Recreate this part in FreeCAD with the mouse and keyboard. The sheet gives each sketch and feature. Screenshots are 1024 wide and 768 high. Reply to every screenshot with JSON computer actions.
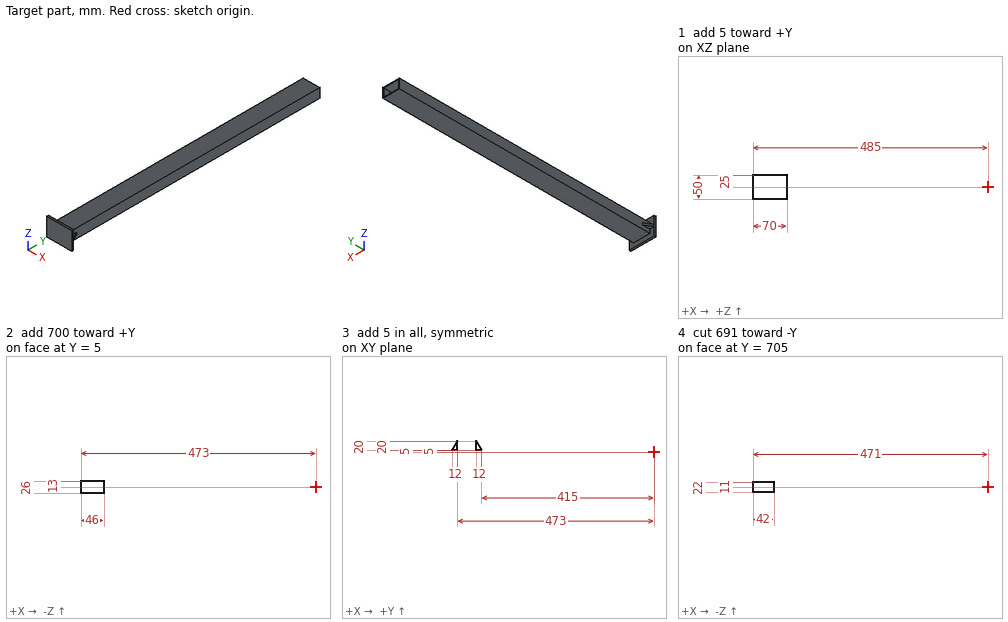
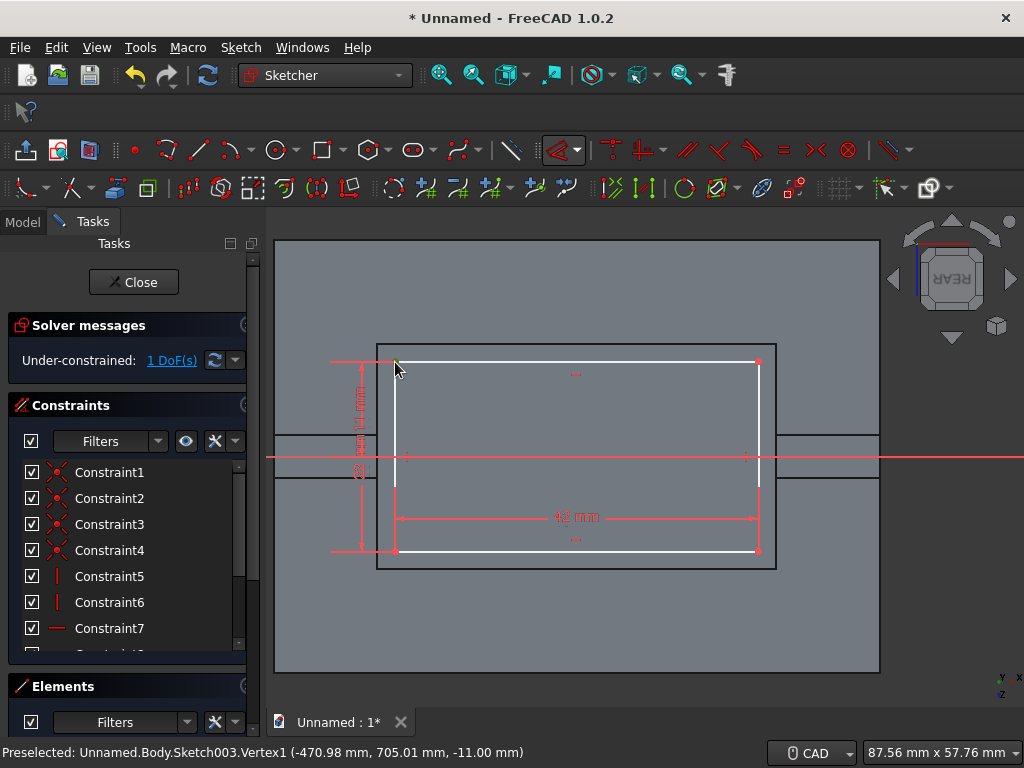
{"action": "key", "text": "l"}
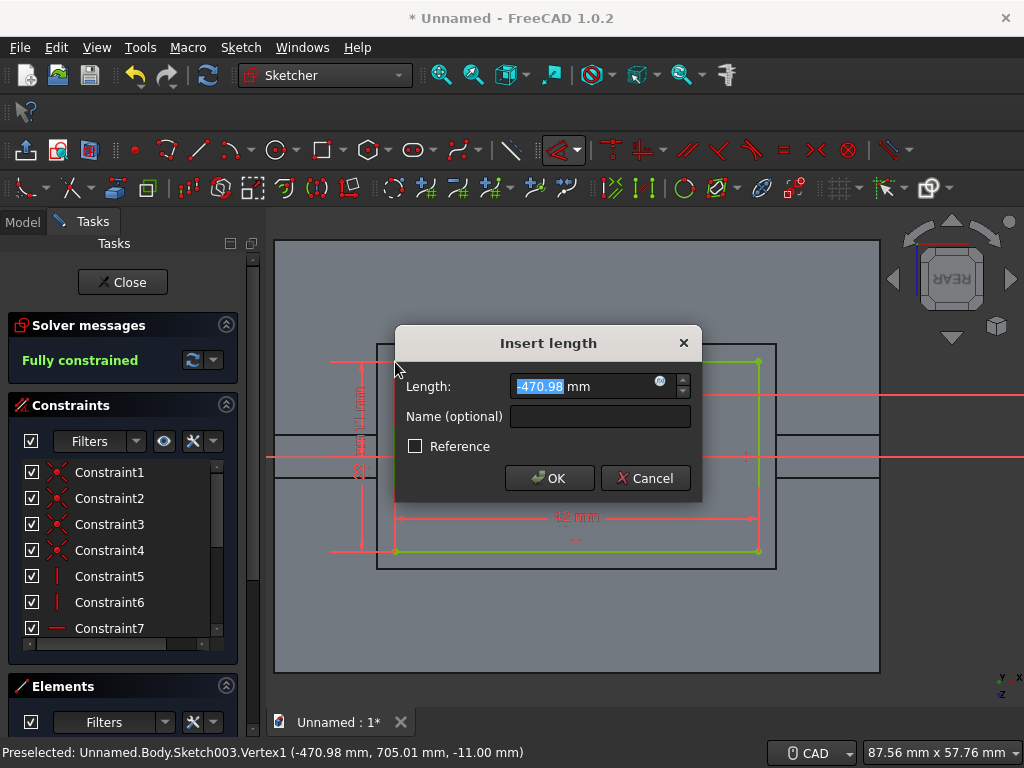
{"action": "type", "text": "-471"}
{"action": "key", "text": "Return"}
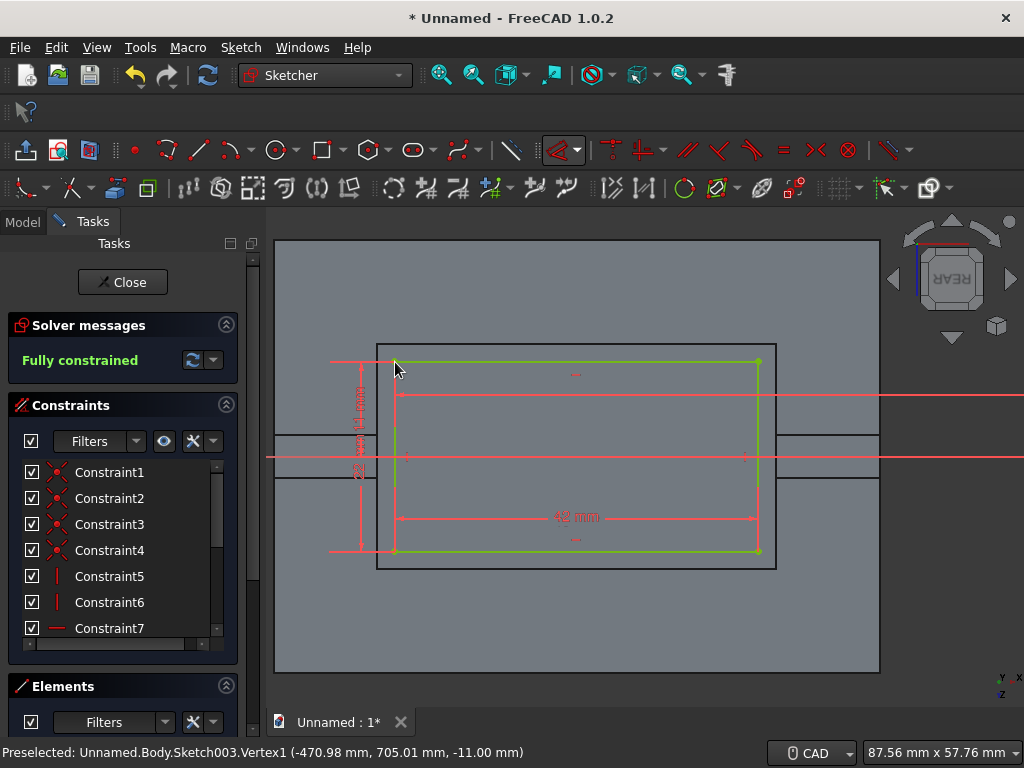
{"action": "left_click", "coordinate": [123, 282]}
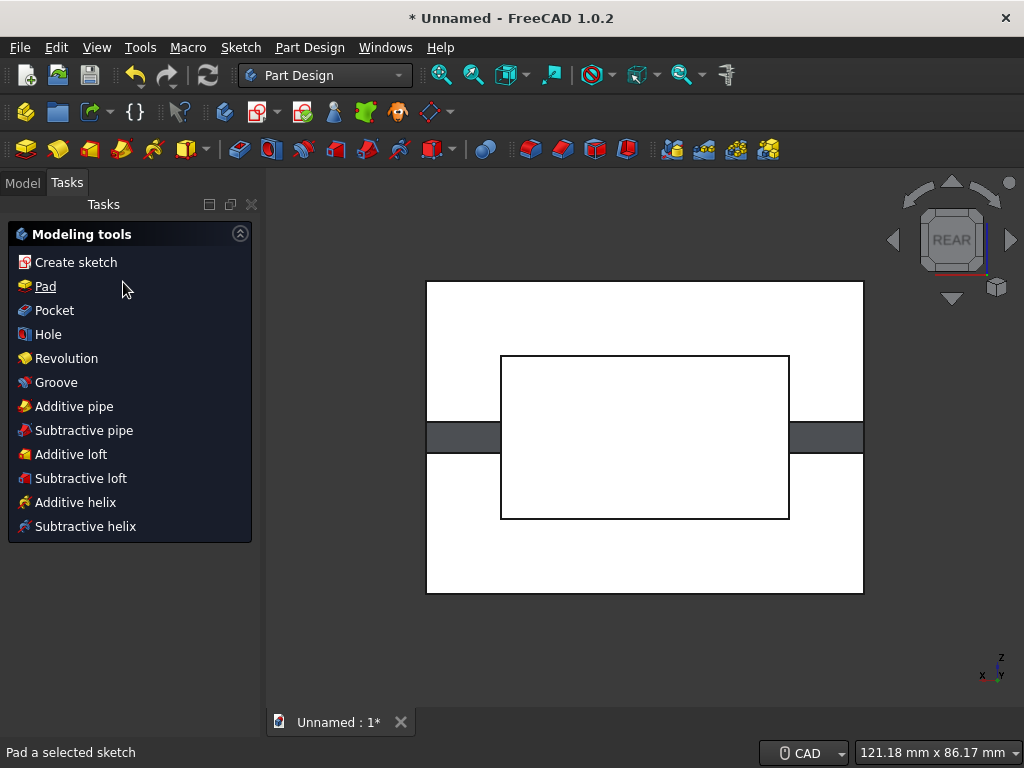
{"action": "left_click", "coordinate": [240, 150]}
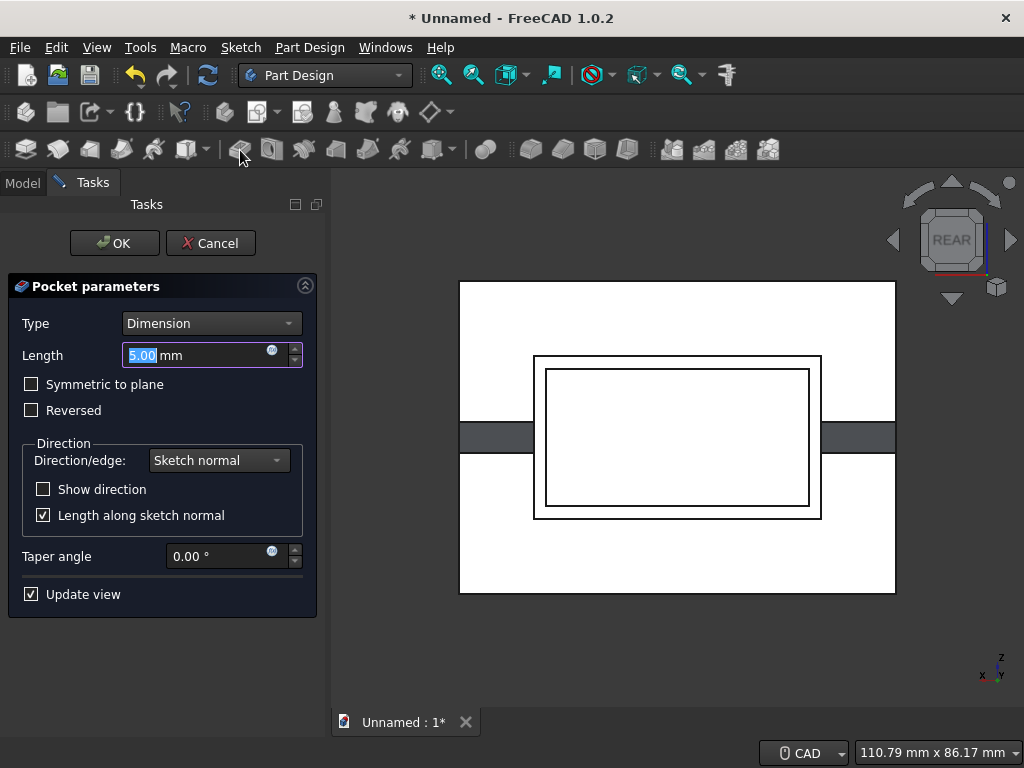
{"action": "type", "text": "691"}
{"action": "key", "text": "Tab"}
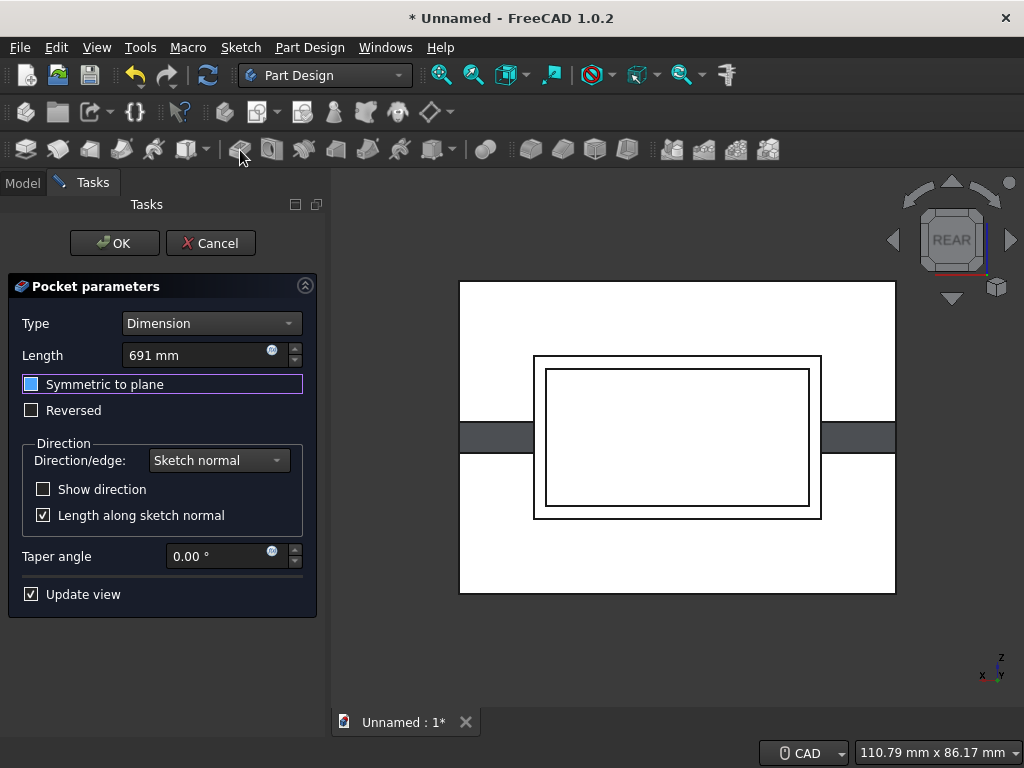
{"action": "left_click", "coordinate": [115, 243]}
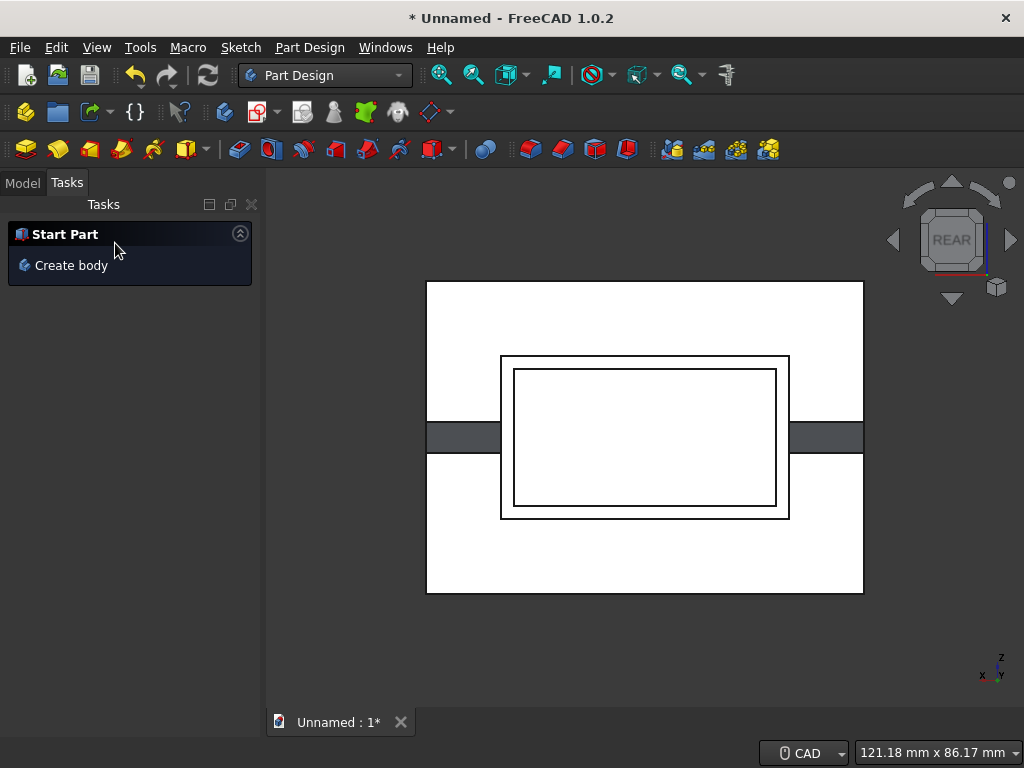
{"action": "key", "text": "0"}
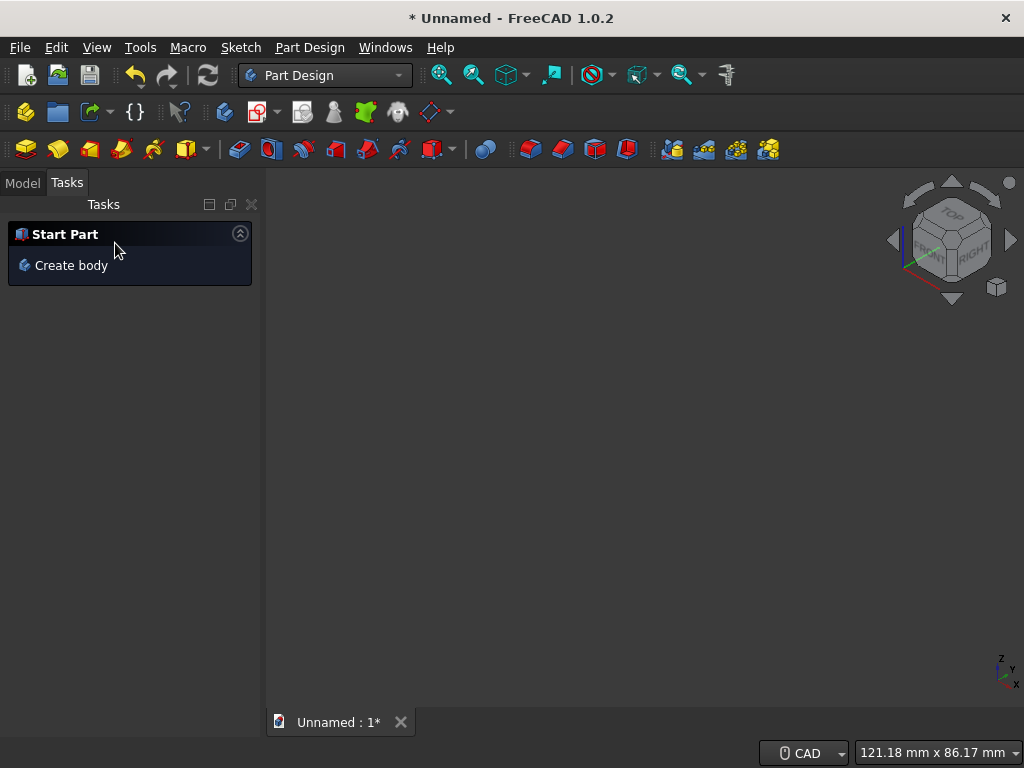
{"action": "key", "text": "v f"}